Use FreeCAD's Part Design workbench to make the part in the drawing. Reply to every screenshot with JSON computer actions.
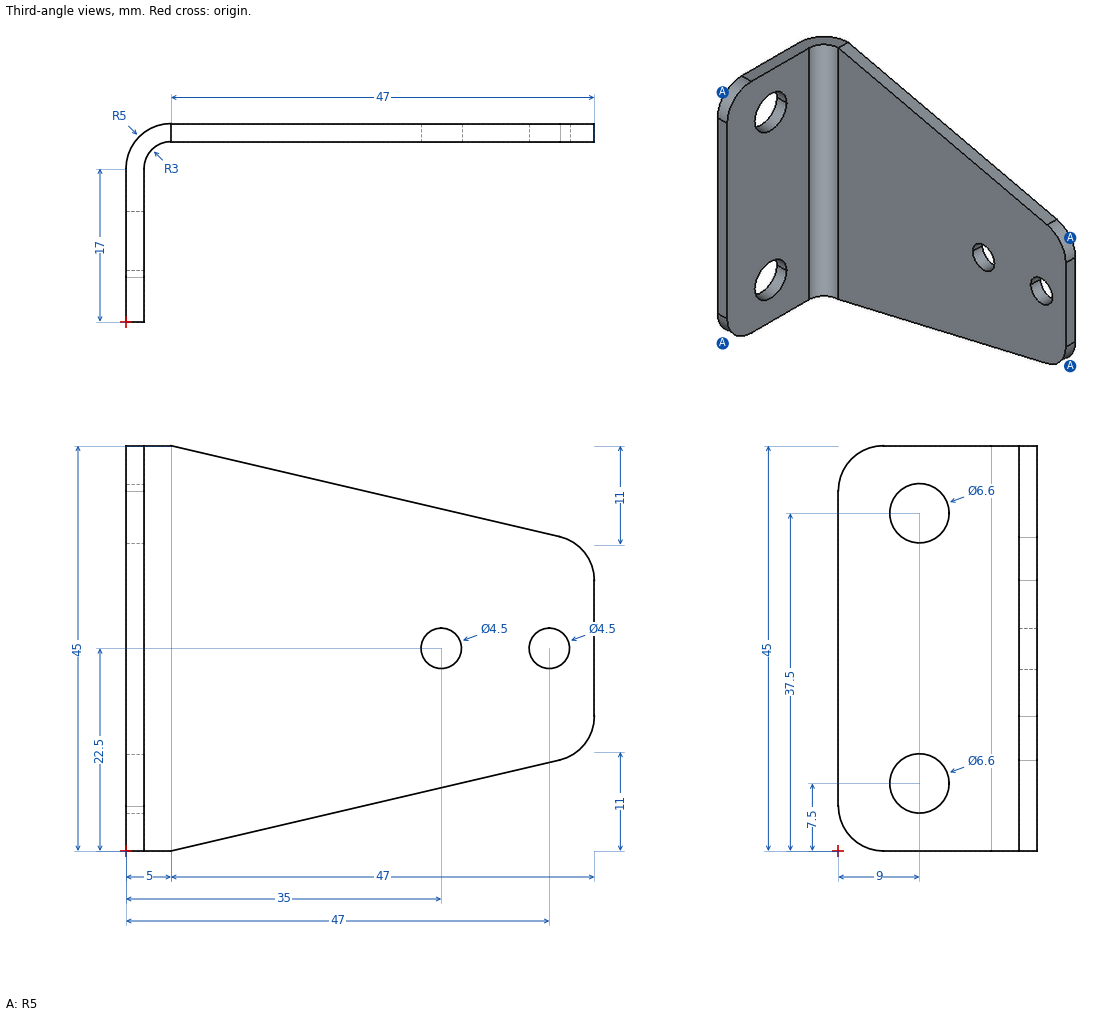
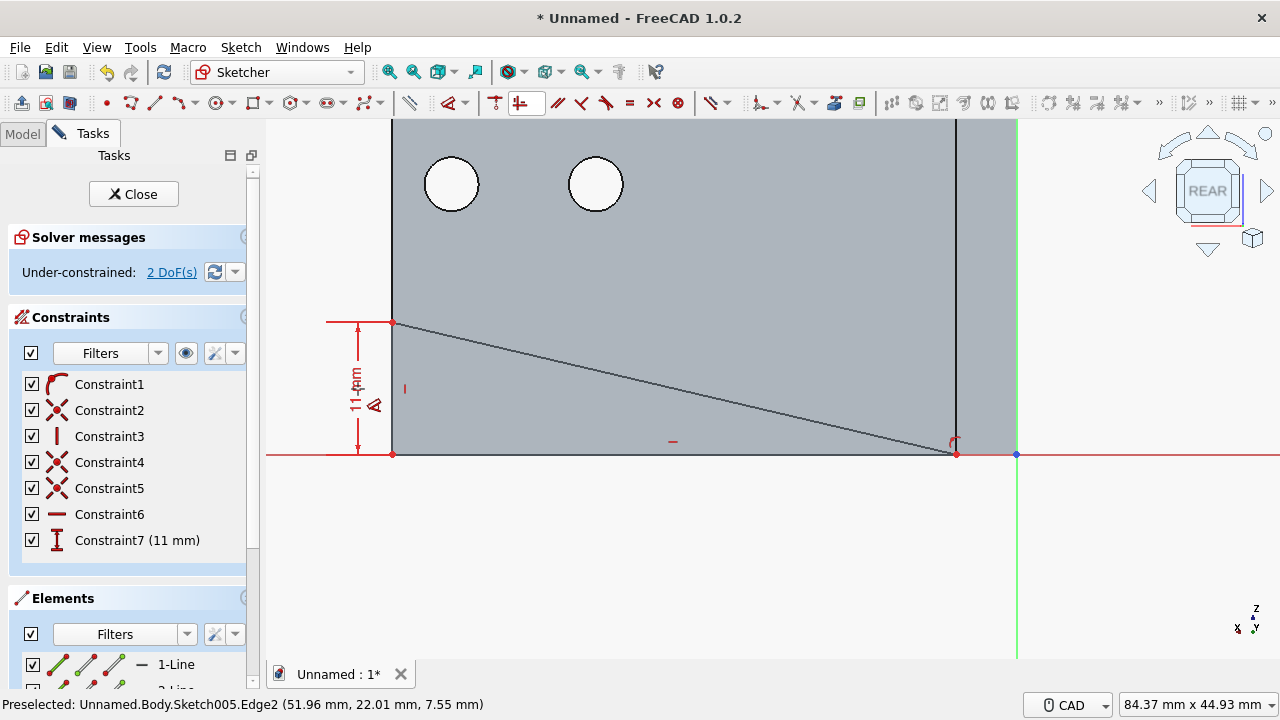
{"action": "left_click", "coordinate": [561, 455]}
{"action": "left_click", "coordinate": [674, 489]}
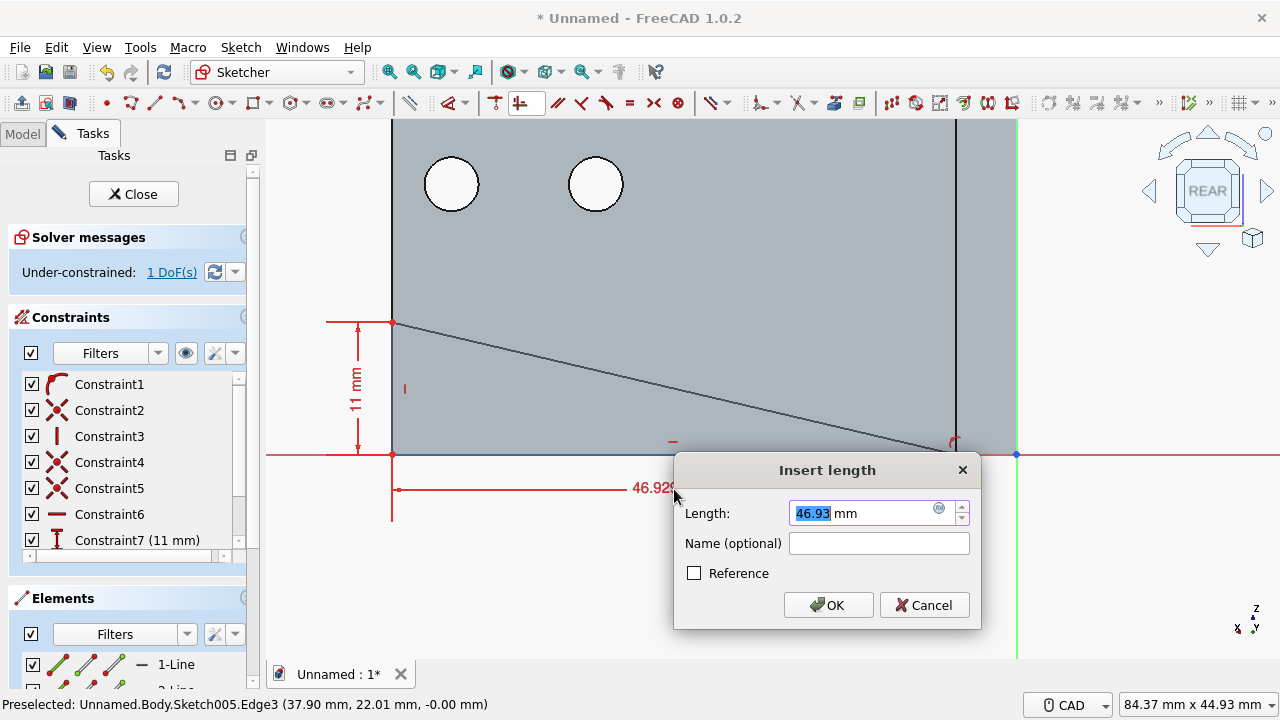
{"action": "type", "text": "47"}
{"action": "key", "text": "Return"}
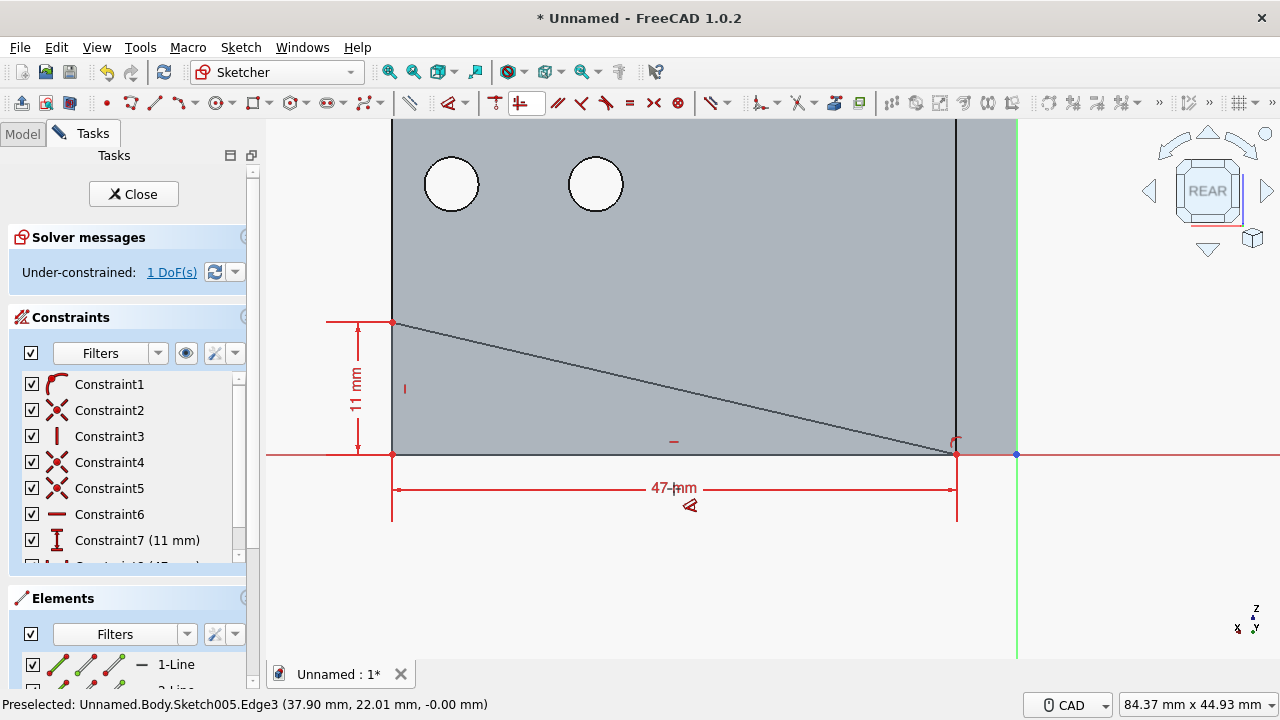
{"action": "left_click", "coordinate": [957, 455]}
{"action": "left_click", "coordinate": [987, 489]}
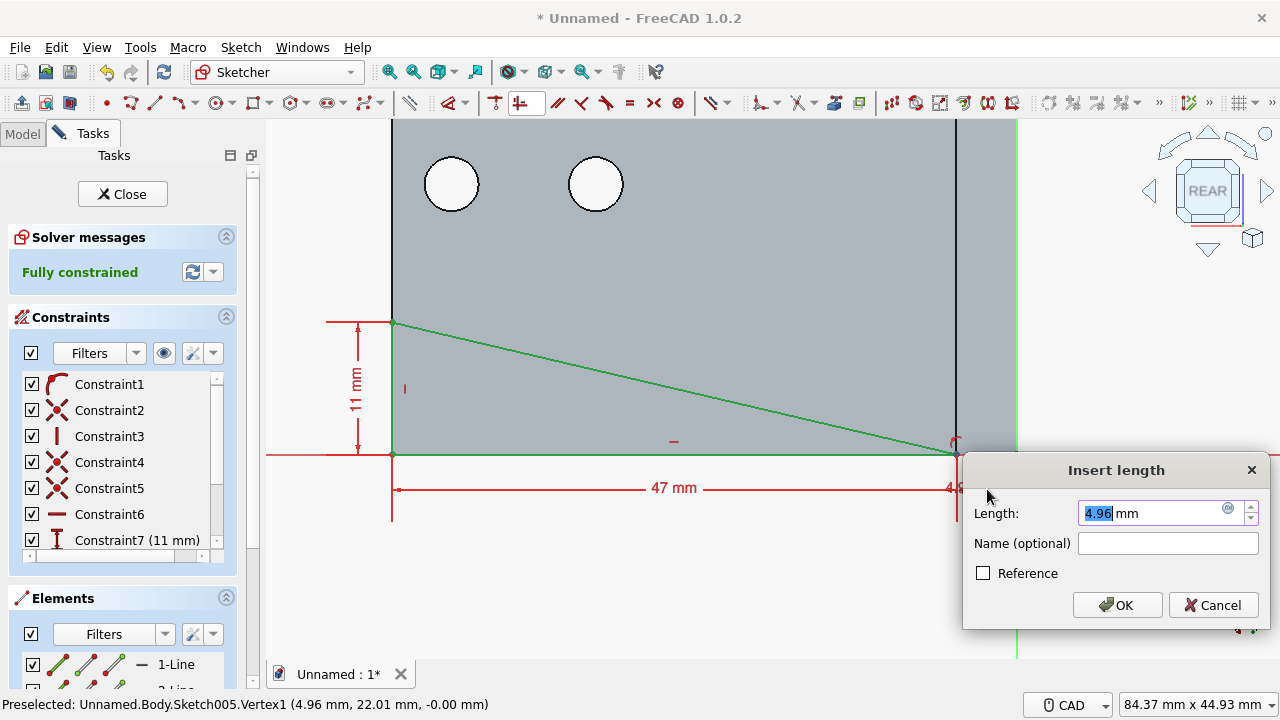
{"action": "type", "text": "5"}
{"action": "key", "text": "Return"}
{"action": "key", "text": "Escape"}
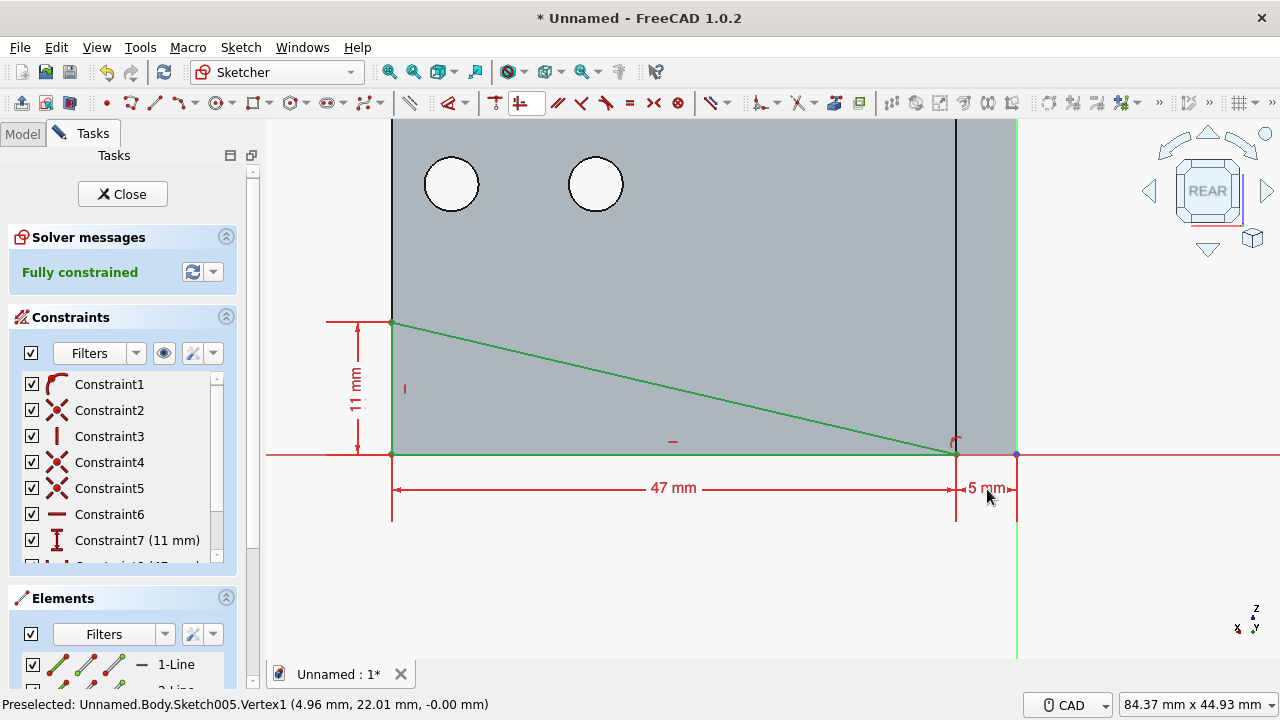
{"action": "left_click", "coordinate": [123, 194]}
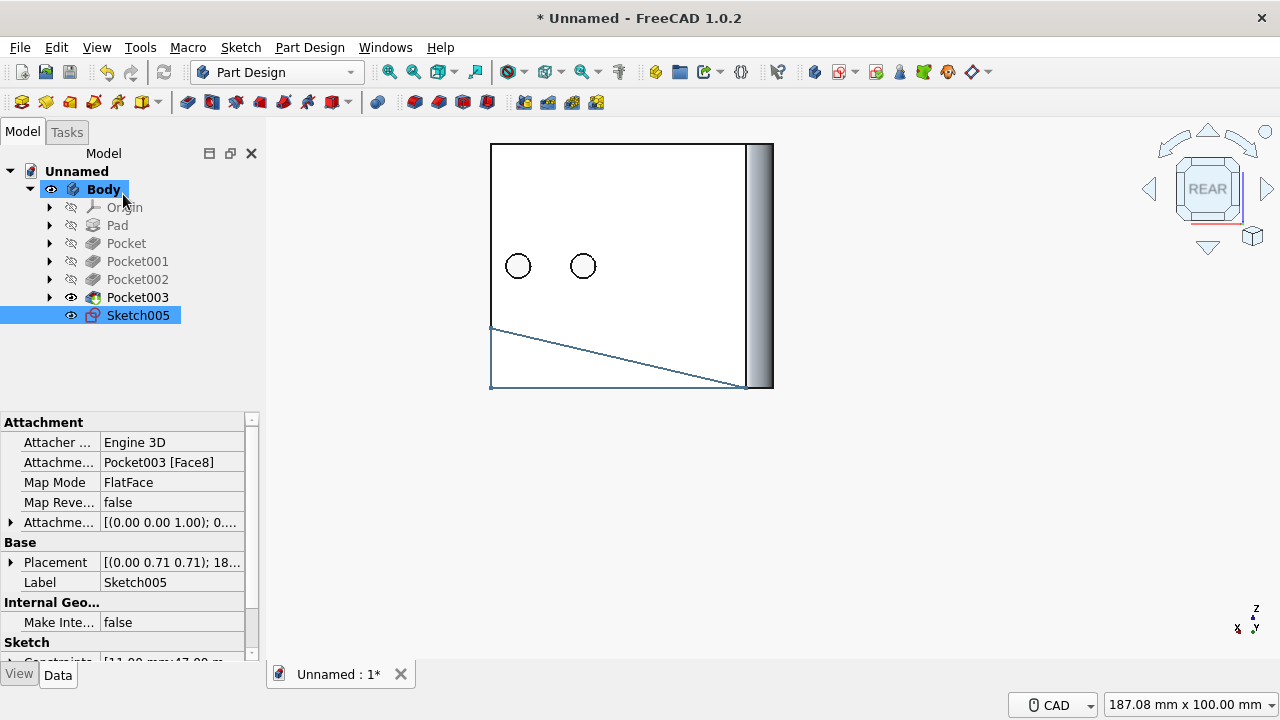
{"action": "left_click", "coordinate": [188, 102]}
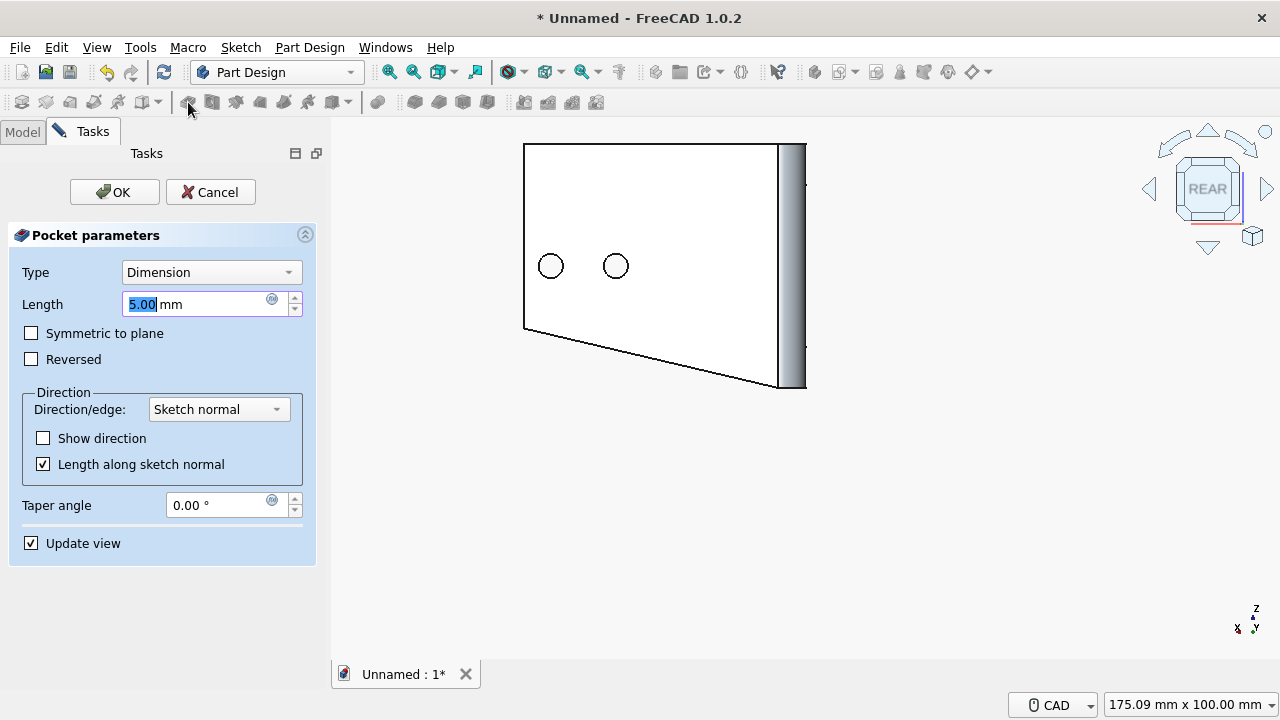
{"action": "left_click", "coordinate": [212, 272]}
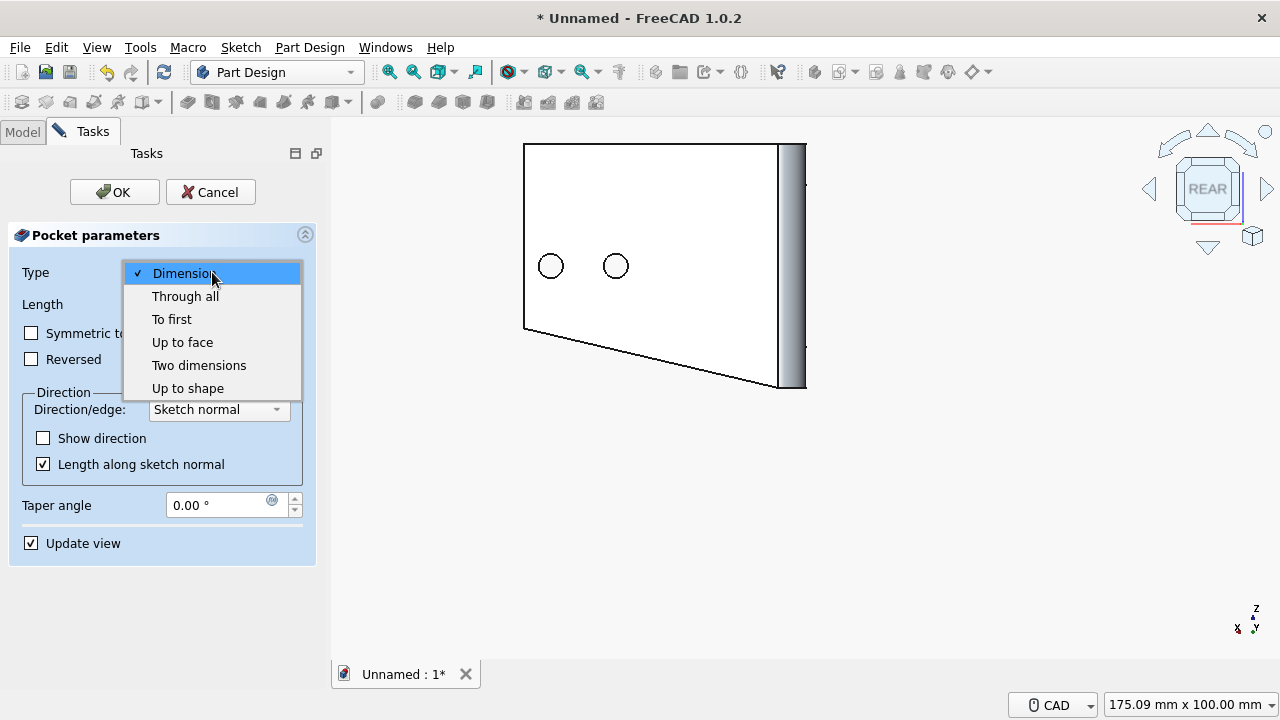
{"action": "left_click", "coordinate": [212, 320]}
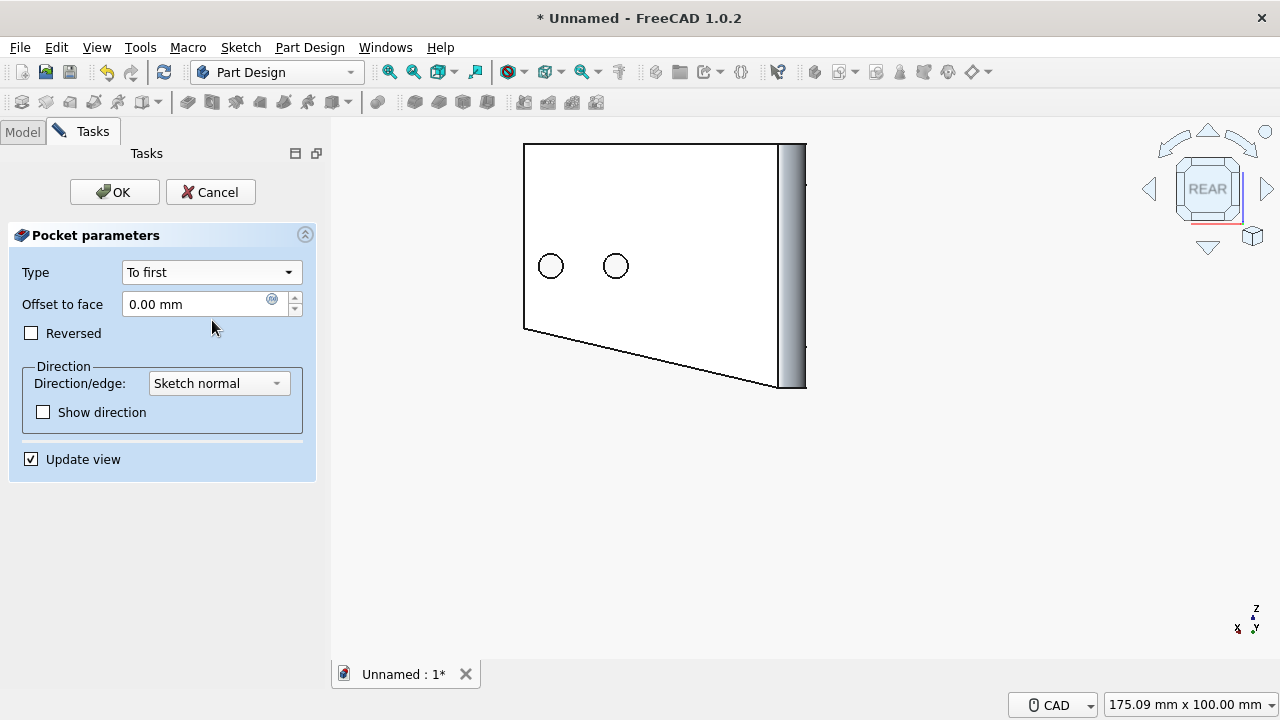
{"action": "left_click", "coordinate": [115, 192]}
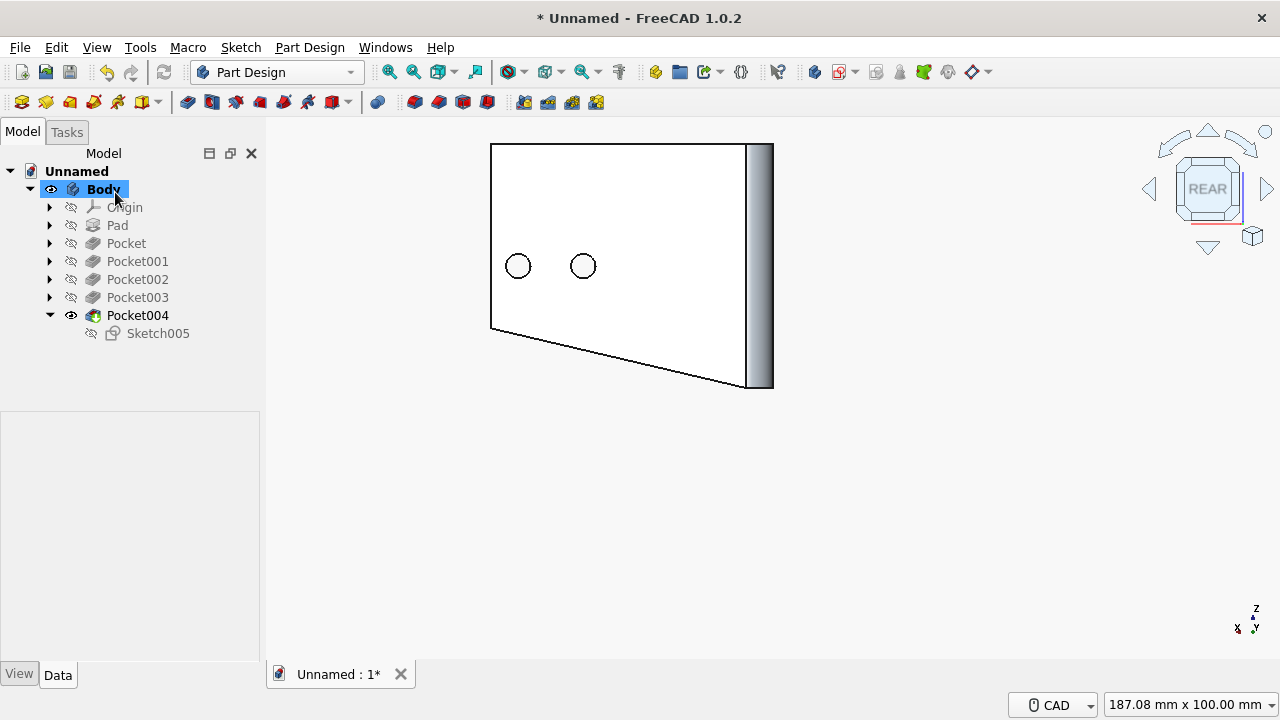
{"action": "left_click", "coordinate": [655, 230]}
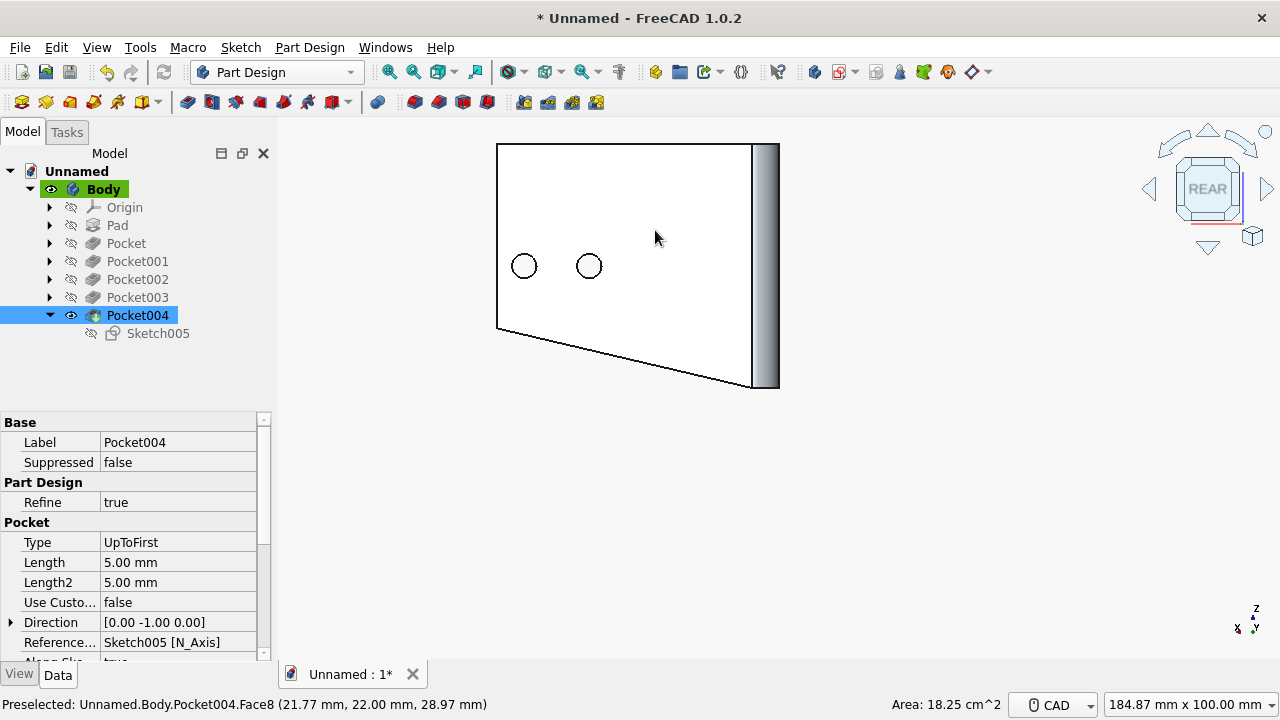
{"action": "left_click", "coordinate": [840, 72]}